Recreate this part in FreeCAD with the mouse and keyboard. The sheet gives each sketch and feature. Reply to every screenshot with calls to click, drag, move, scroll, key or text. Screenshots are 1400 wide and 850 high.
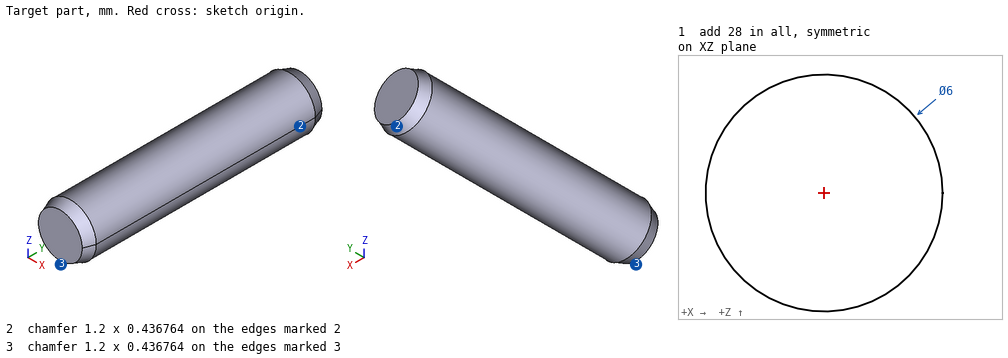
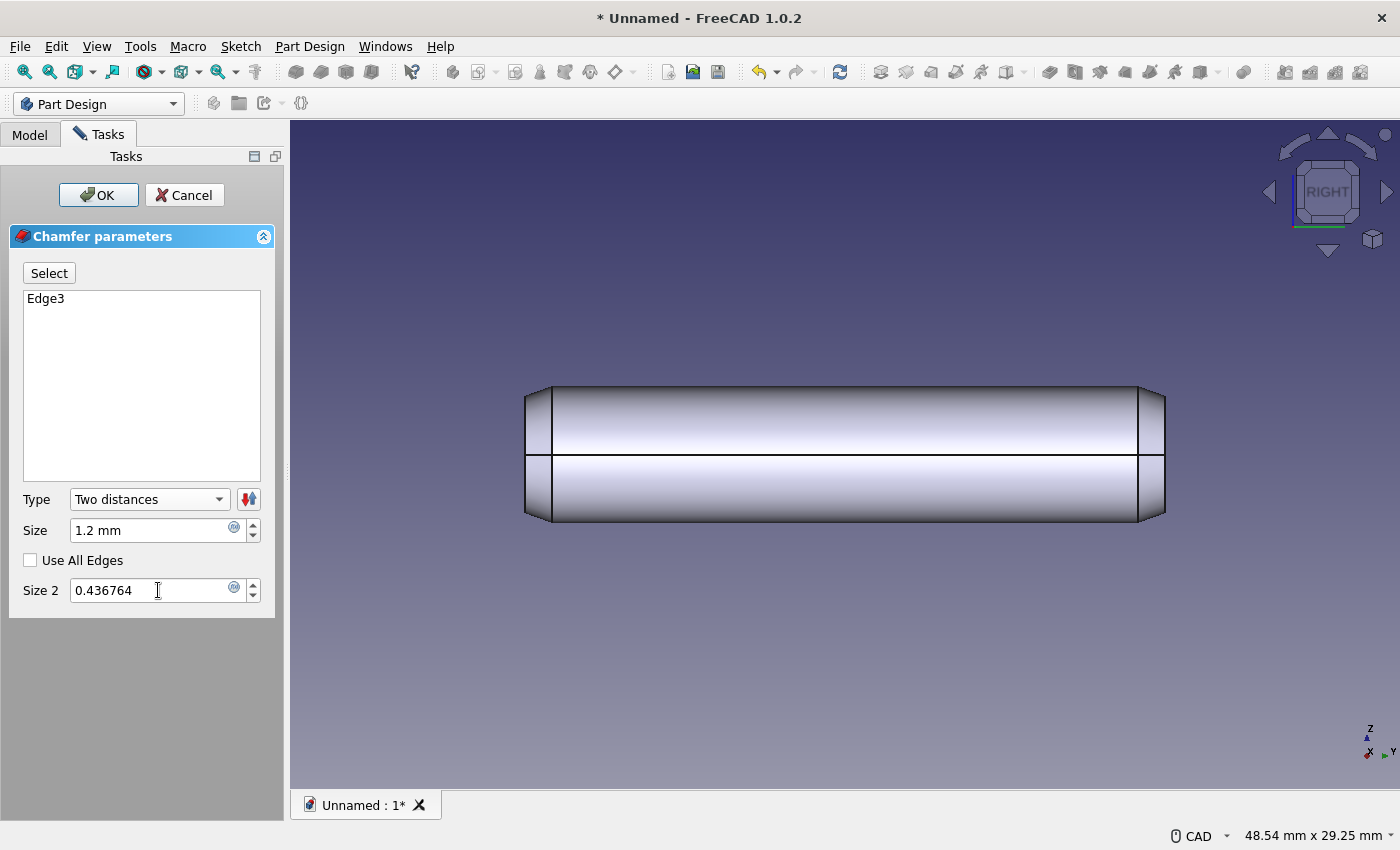
click(99, 195)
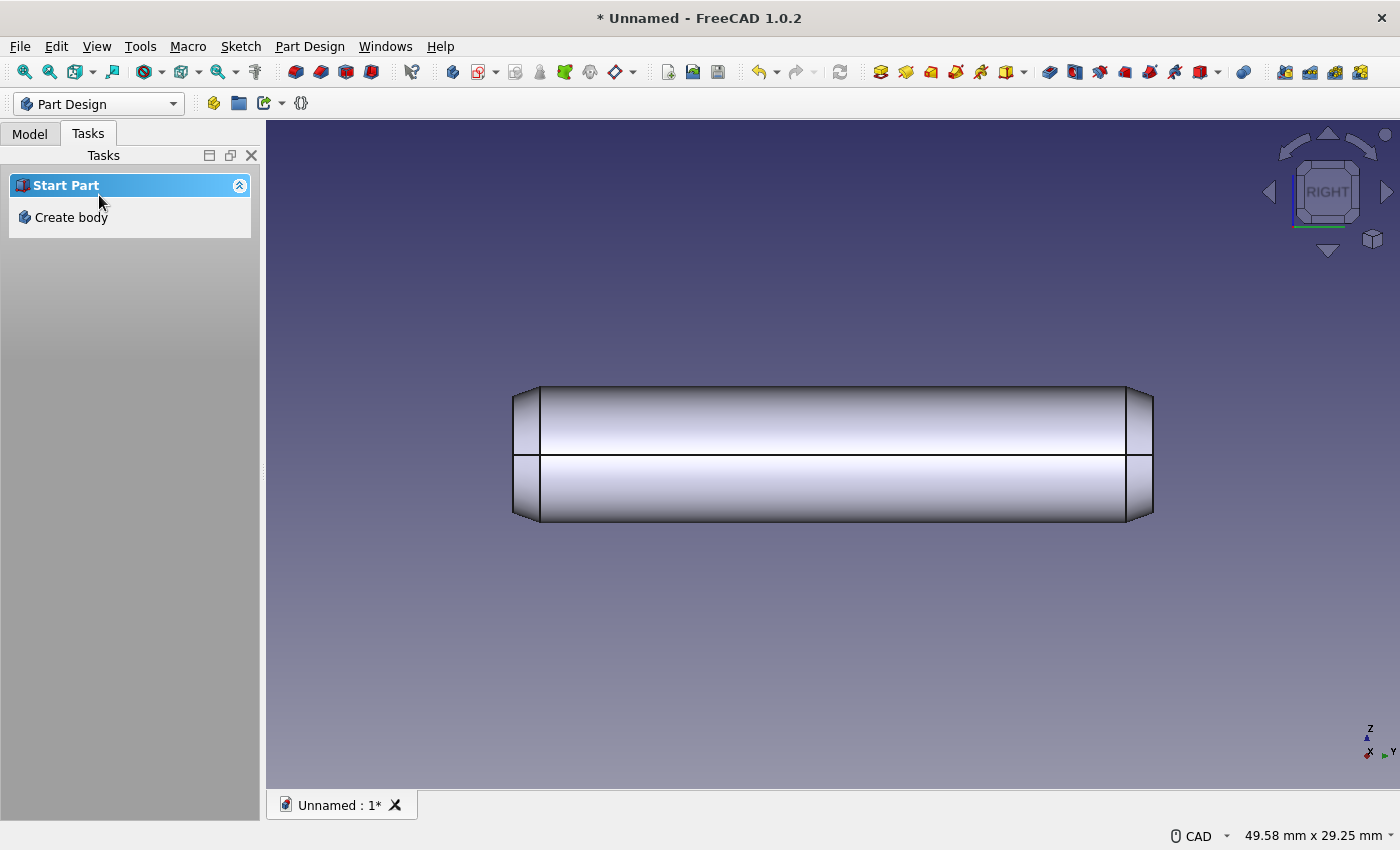
key(0)